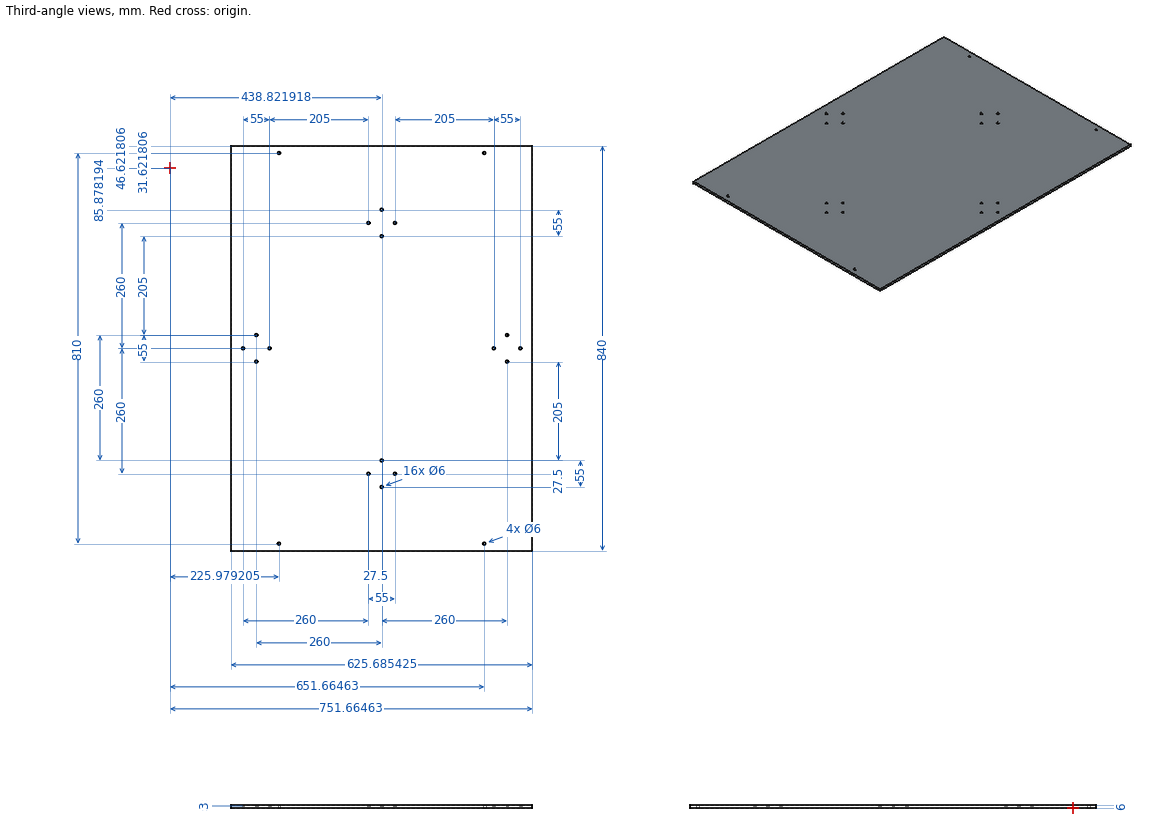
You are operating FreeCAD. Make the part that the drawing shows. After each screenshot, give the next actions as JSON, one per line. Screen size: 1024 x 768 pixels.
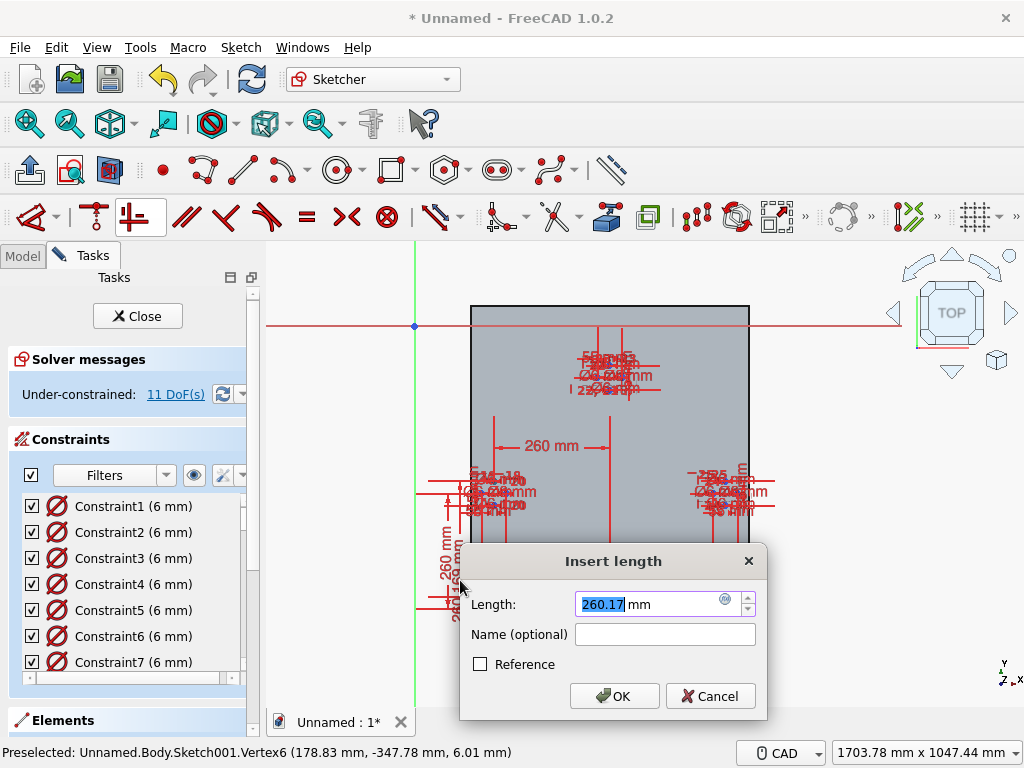
{"action": "type", "text": "260"}
{"action": "key", "text": "Return"}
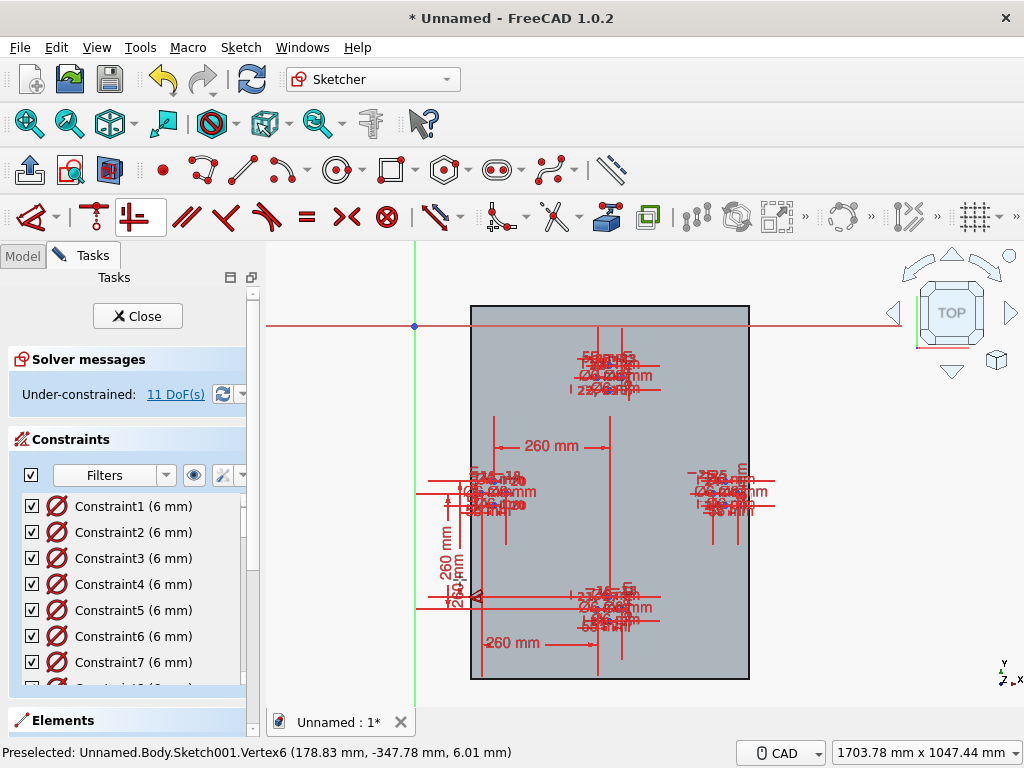
{"action": "left_click", "coordinate": [494, 481]}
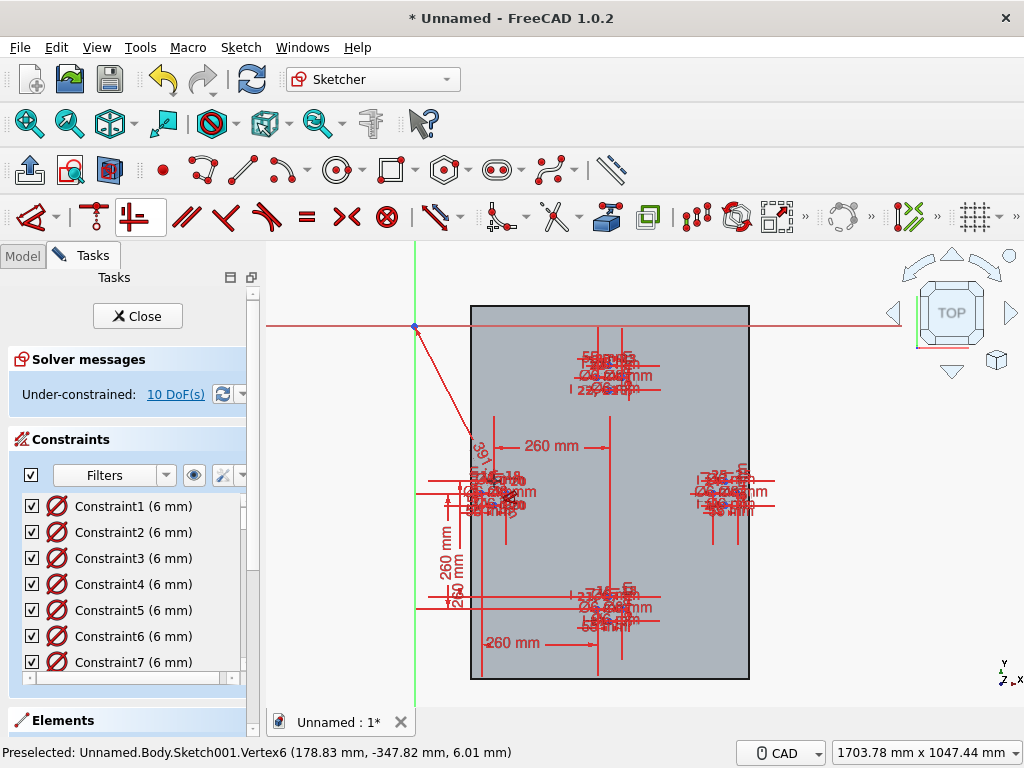
{"action": "left_click", "coordinate": [610, 390]}
{"action": "left_click", "coordinate": [460, 436]}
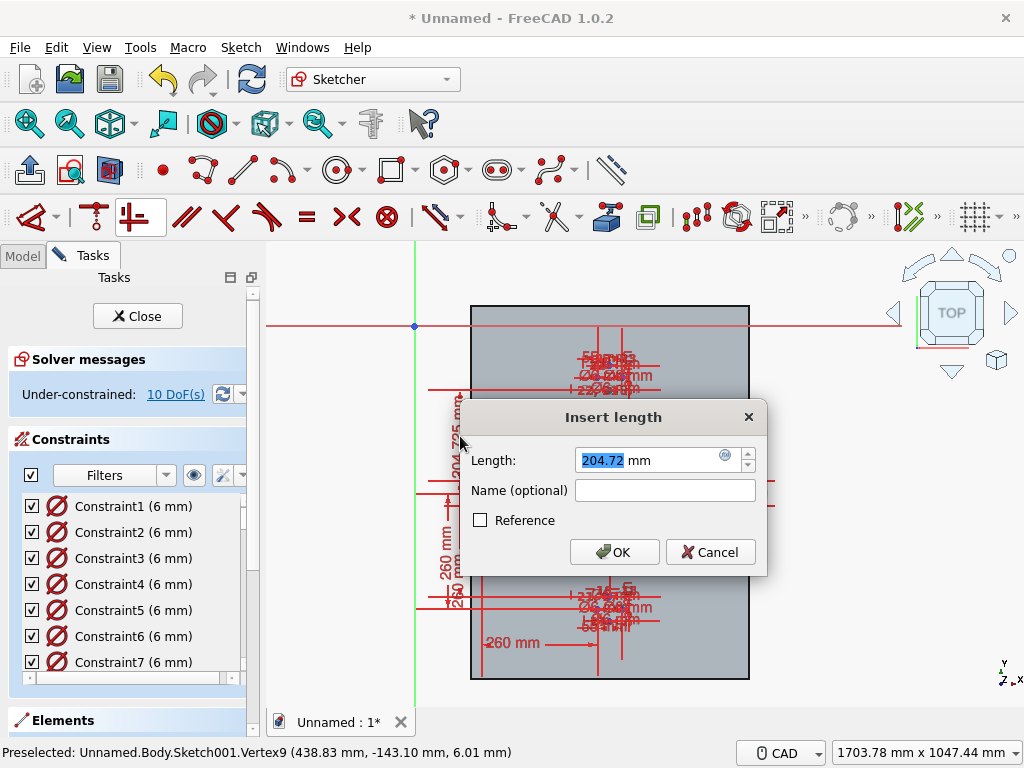
{"action": "type", "text": "205"}
{"action": "key", "text": "Return"}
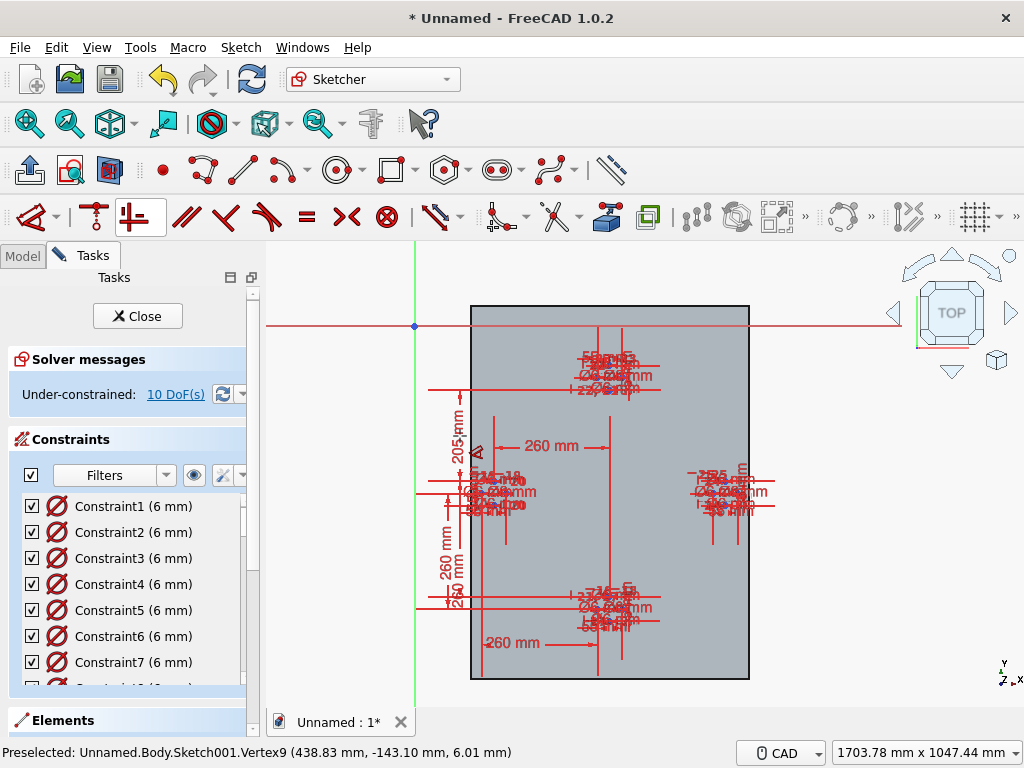
{"action": "left_click", "coordinate": [506, 494]}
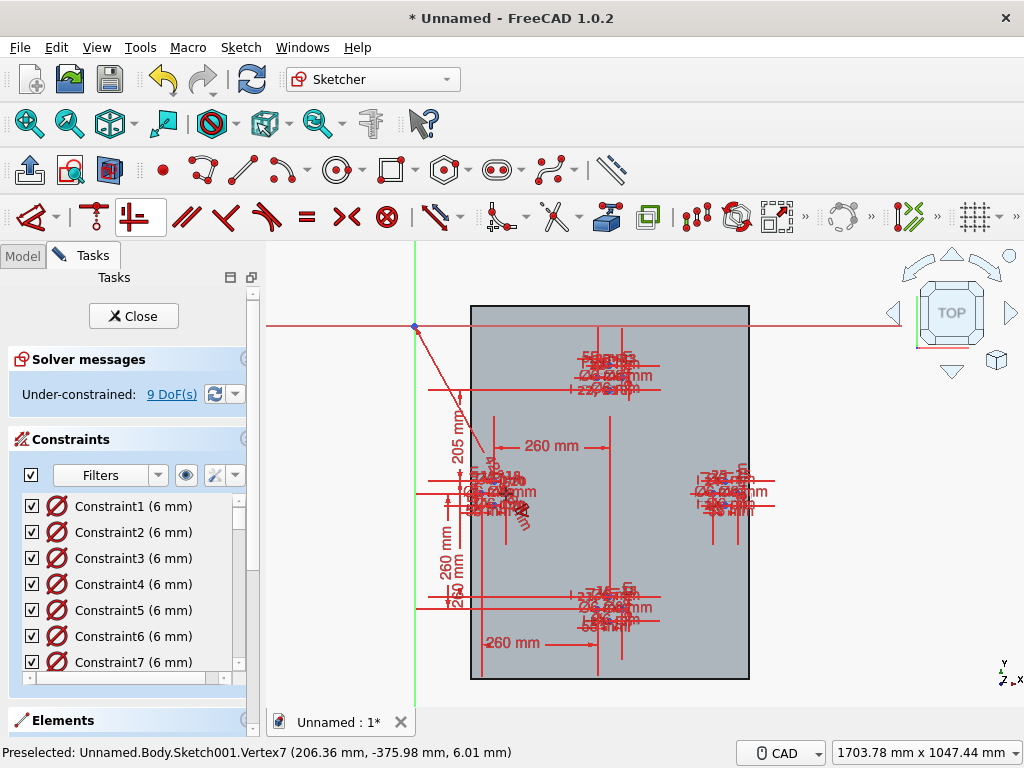
{"action": "left_click", "coordinate": [598, 378]}
{"action": "left_click", "coordinate": [531, 344]}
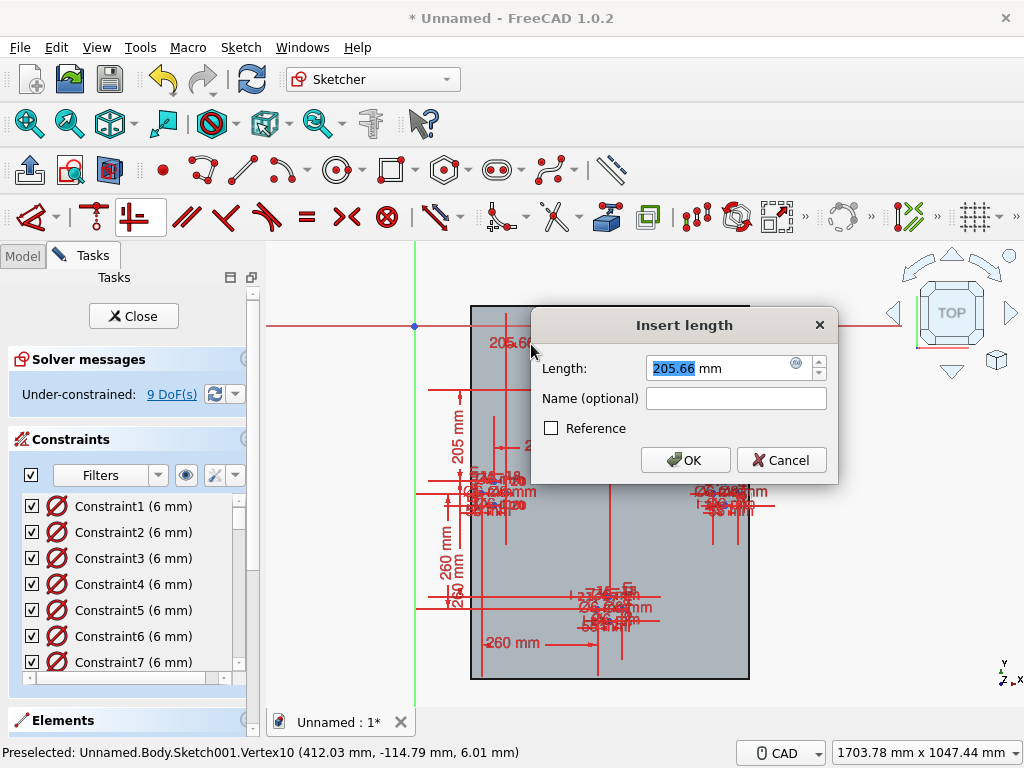
{"action": "type", "text": "205"}
{"action": "key", "text": "Return"}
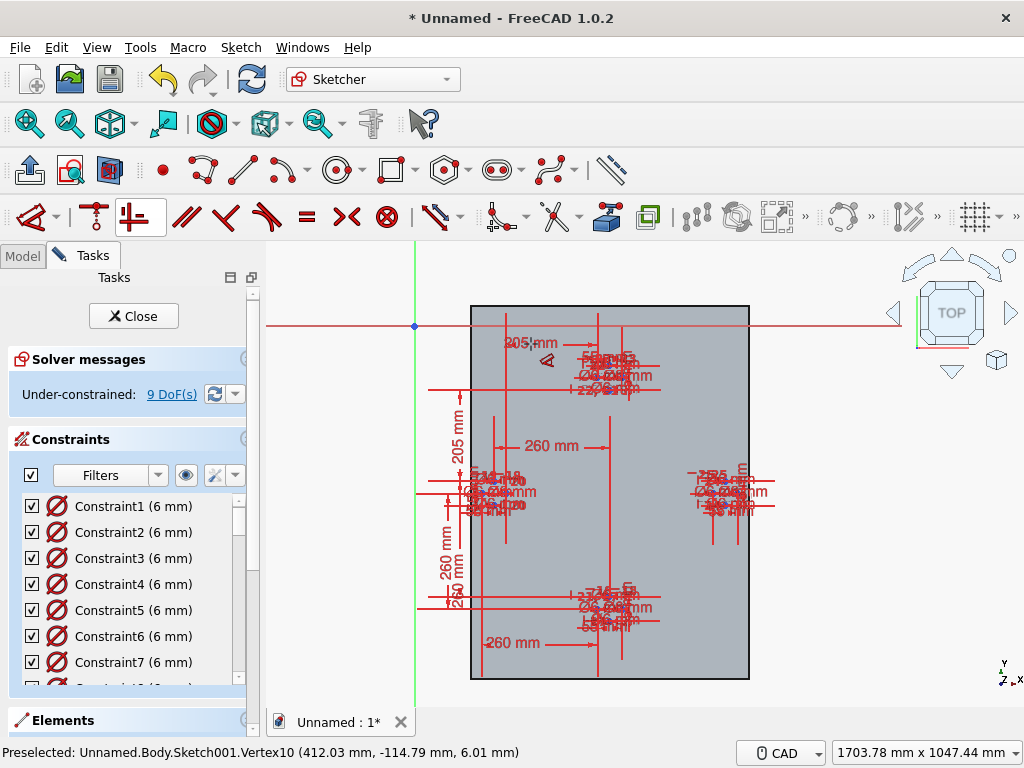
{"action": "left_click", "coordinate": [506, 494]}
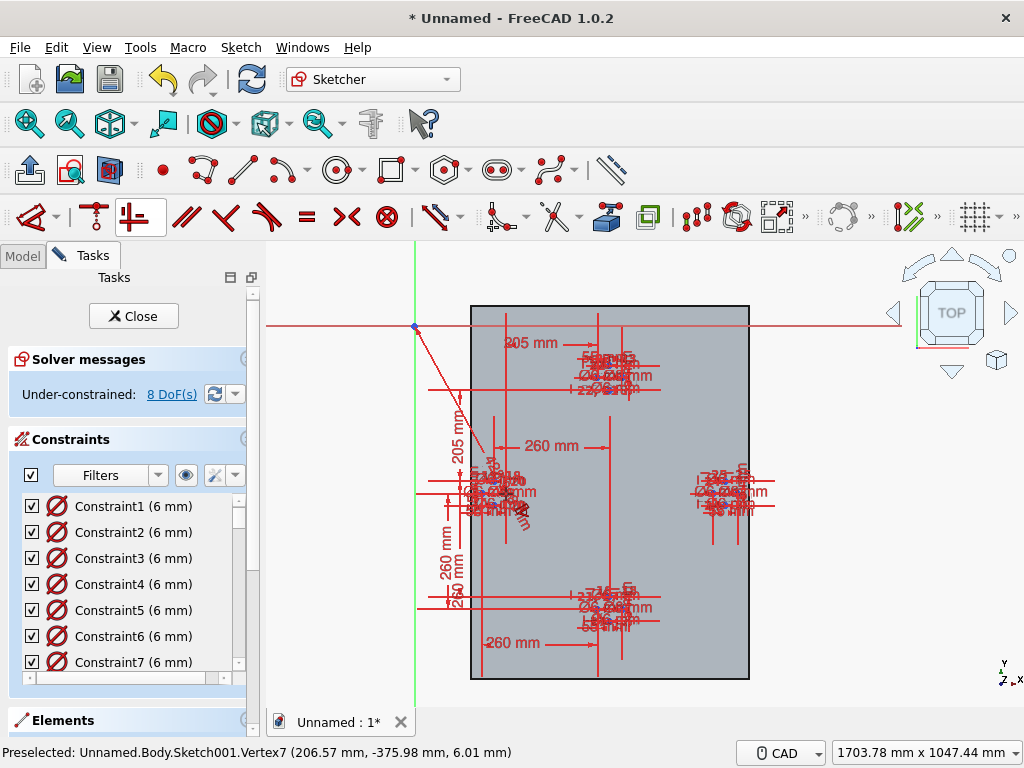
{"action": "left_click", "coordinate": [598, 378]}
{"action": "left_click", "coordinate": [472, 409]}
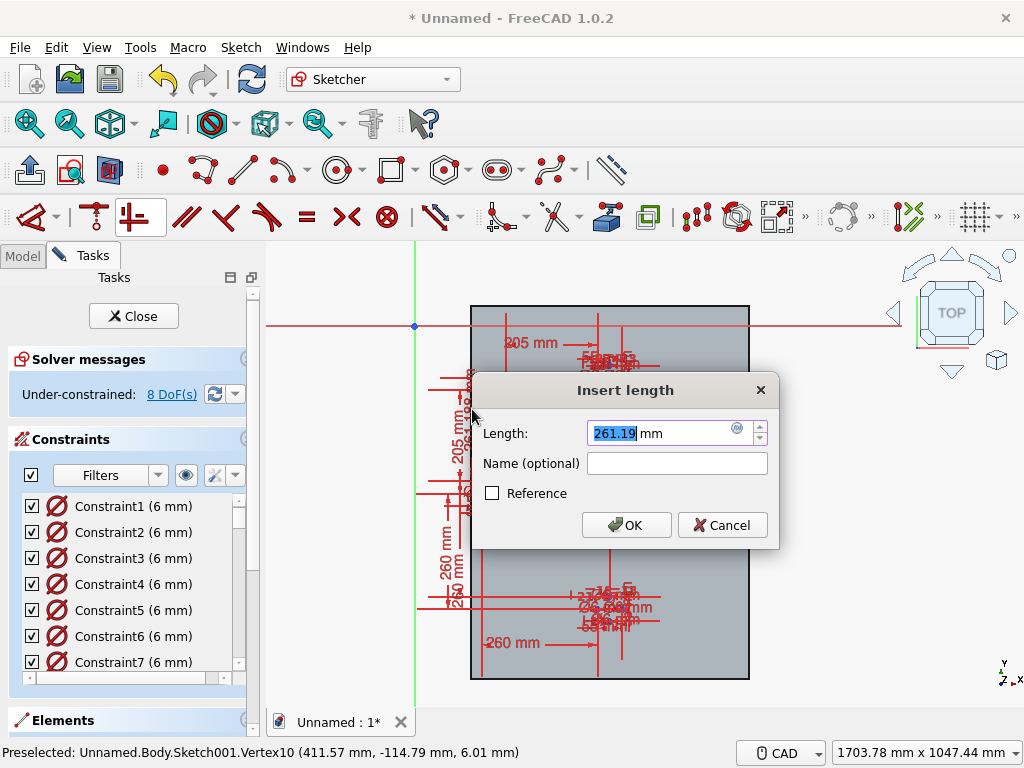
{"action": "type", "text": "260"}
{"action": "key", "text": "Return"}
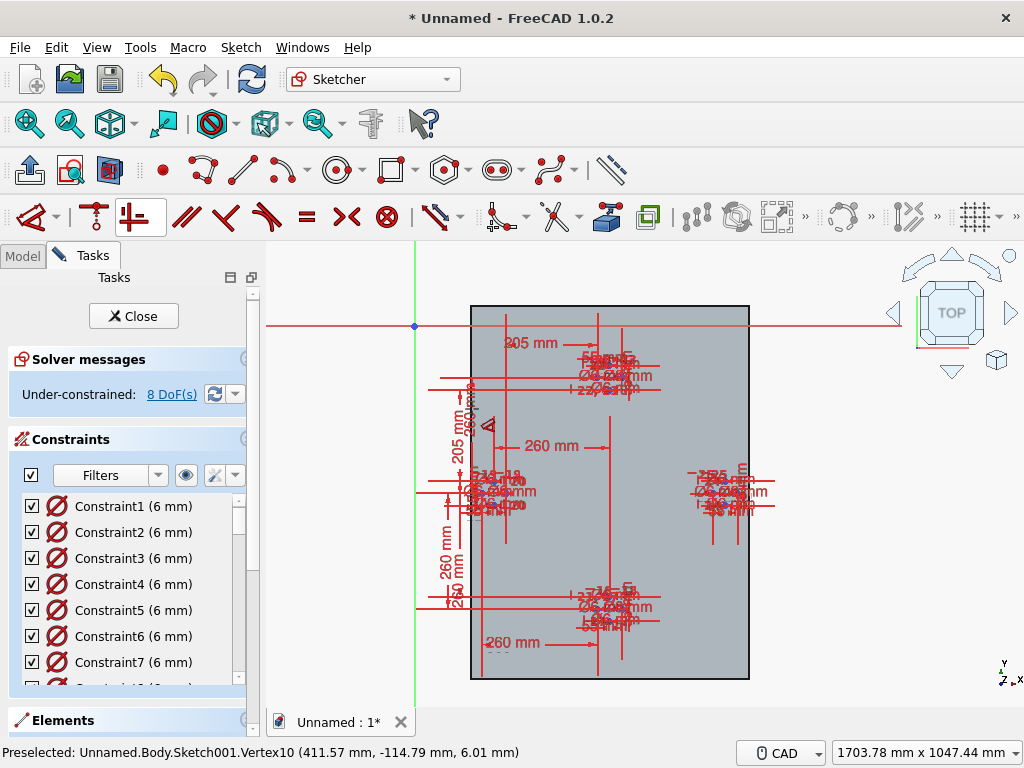
{"action": "left_click", "coordinate": [610, 597]}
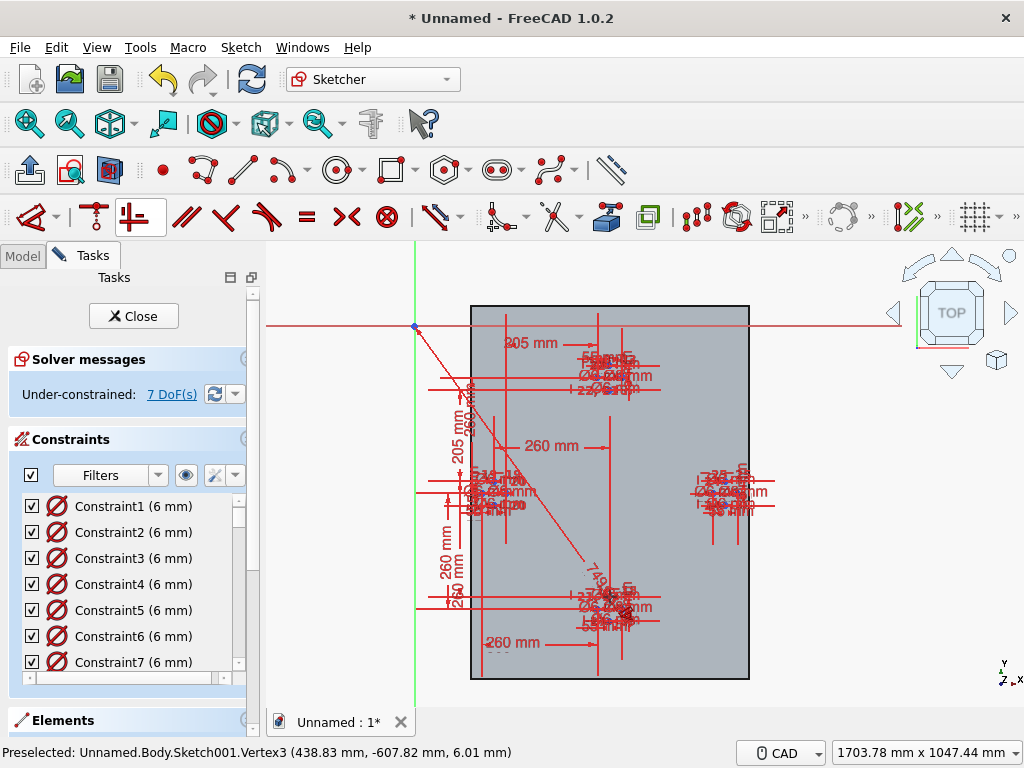
{"action": "left_click", "coordinate": [725, 506]}
{"action": "left_click", "coordinate": [694, 631]}